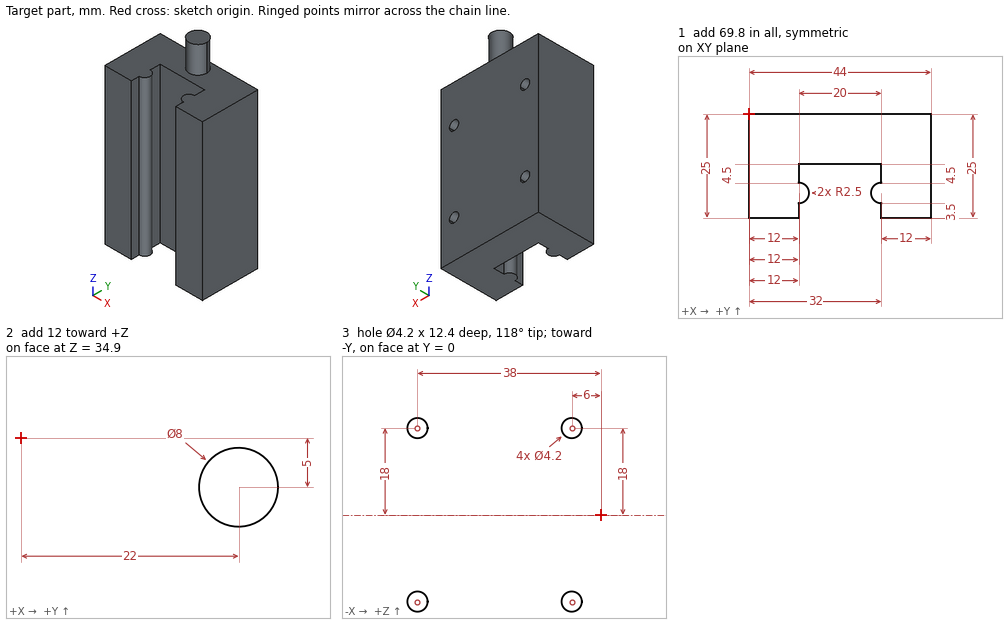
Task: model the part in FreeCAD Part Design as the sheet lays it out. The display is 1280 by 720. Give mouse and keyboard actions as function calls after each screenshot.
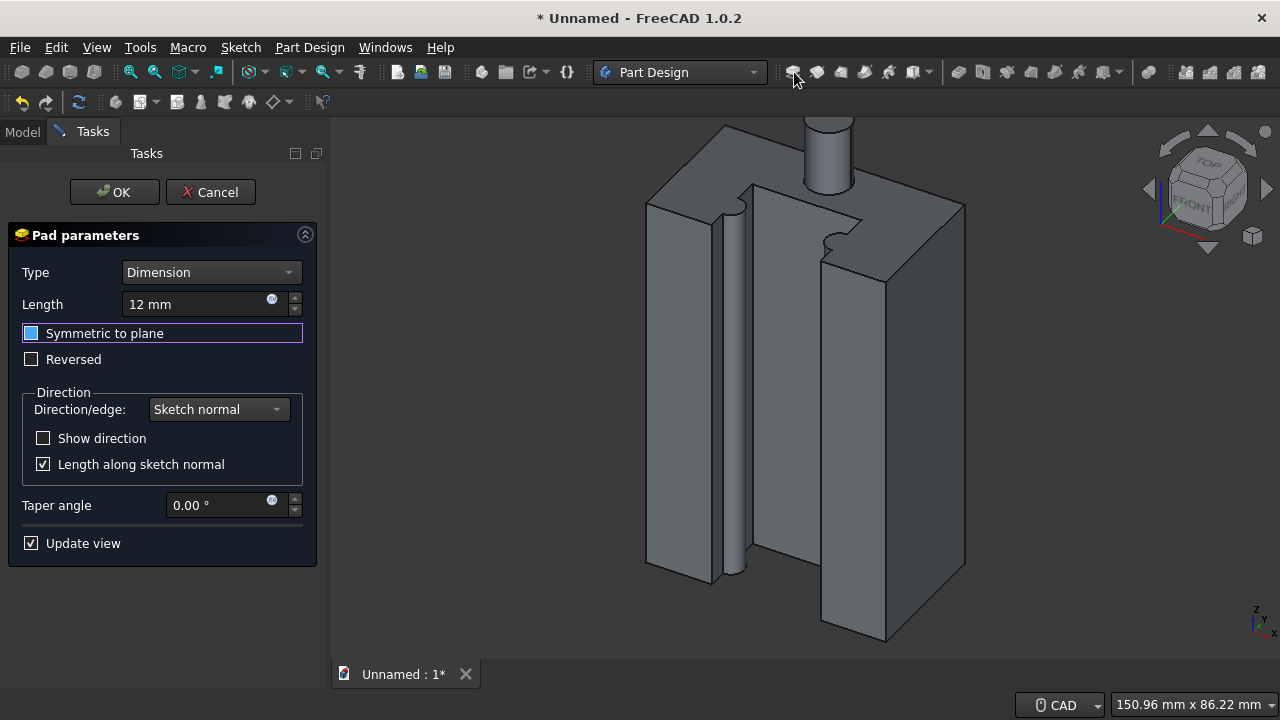
click(115, 192)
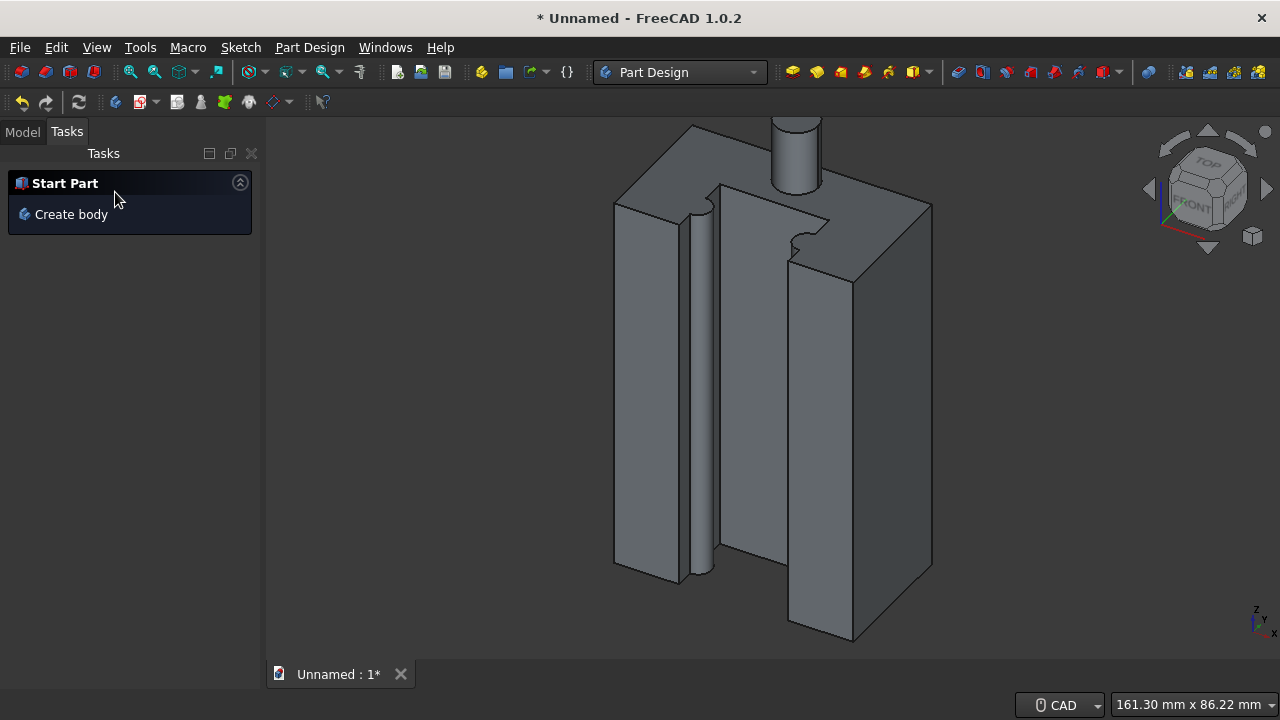
click(132, 72)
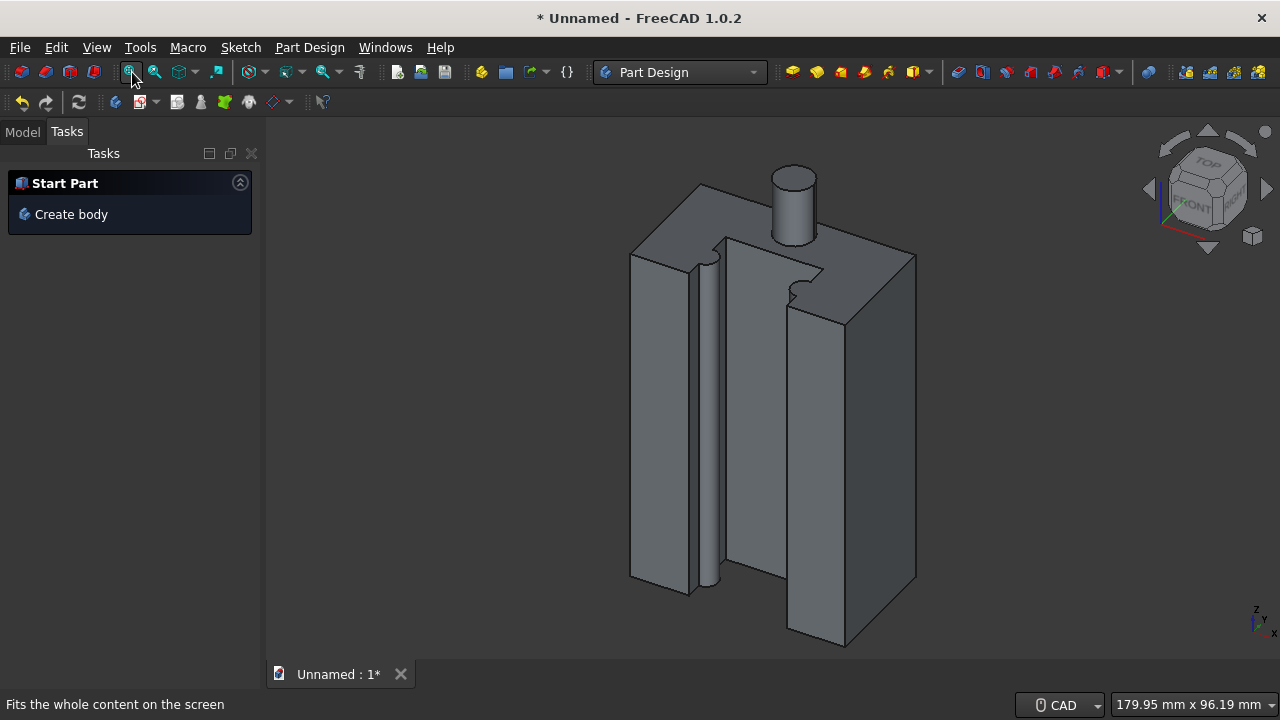
key(4)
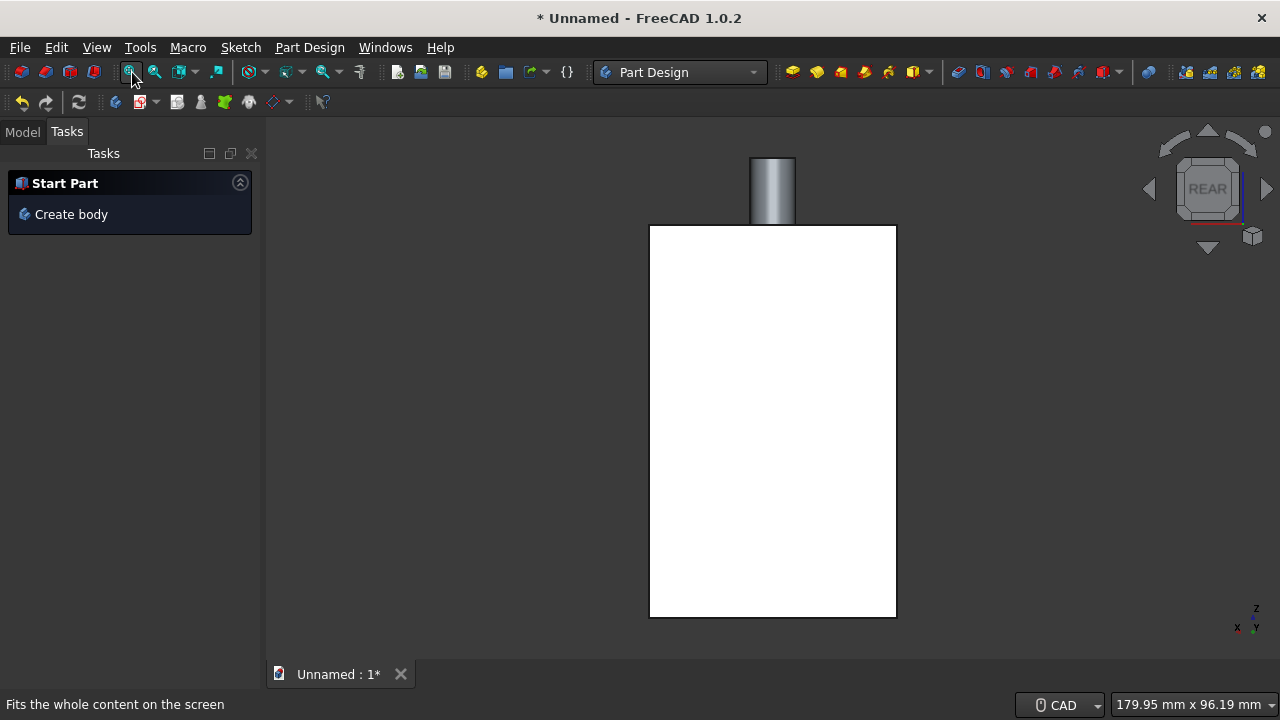
click(773, 365)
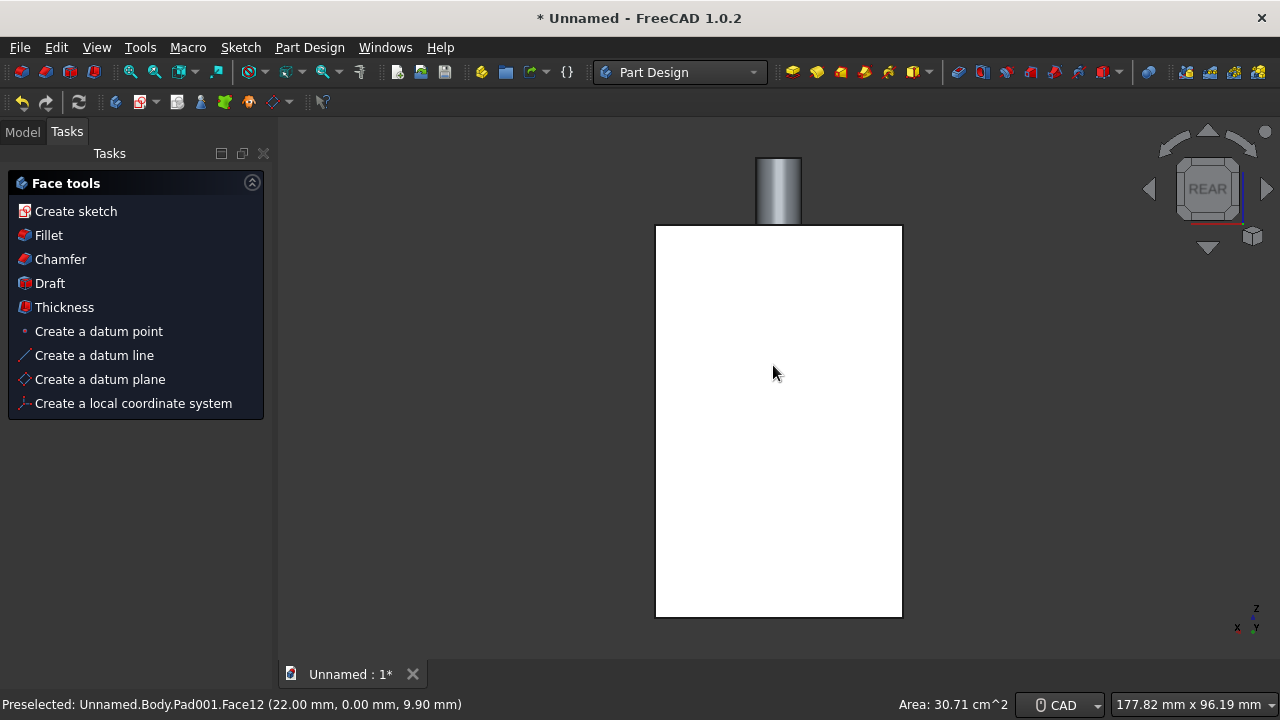
click(140, 102)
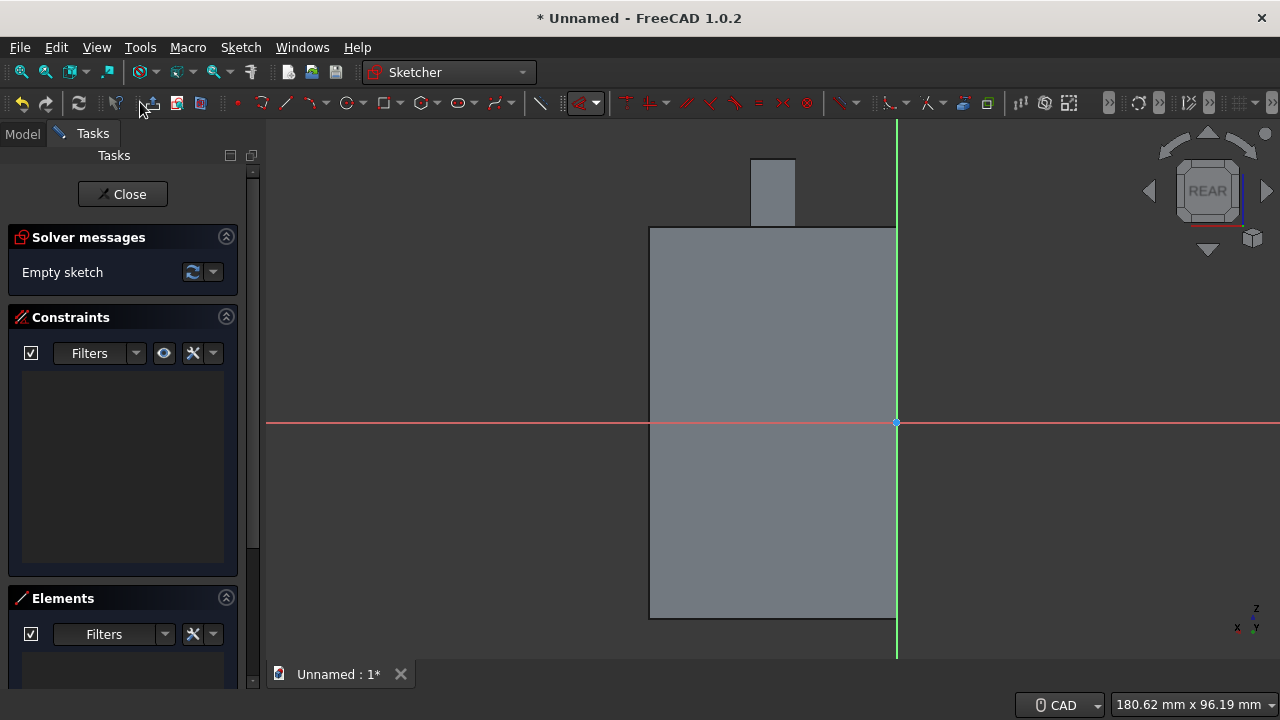
scroll(945, 491, up, 2)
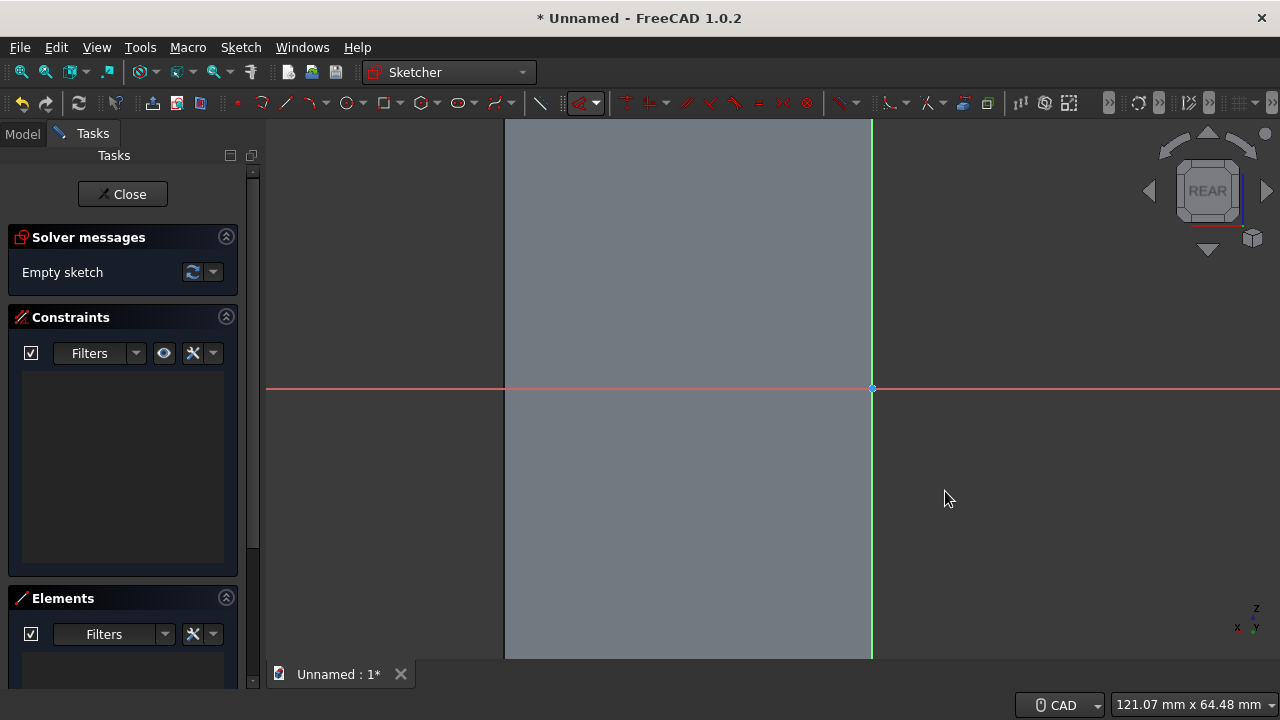
click(348, 104)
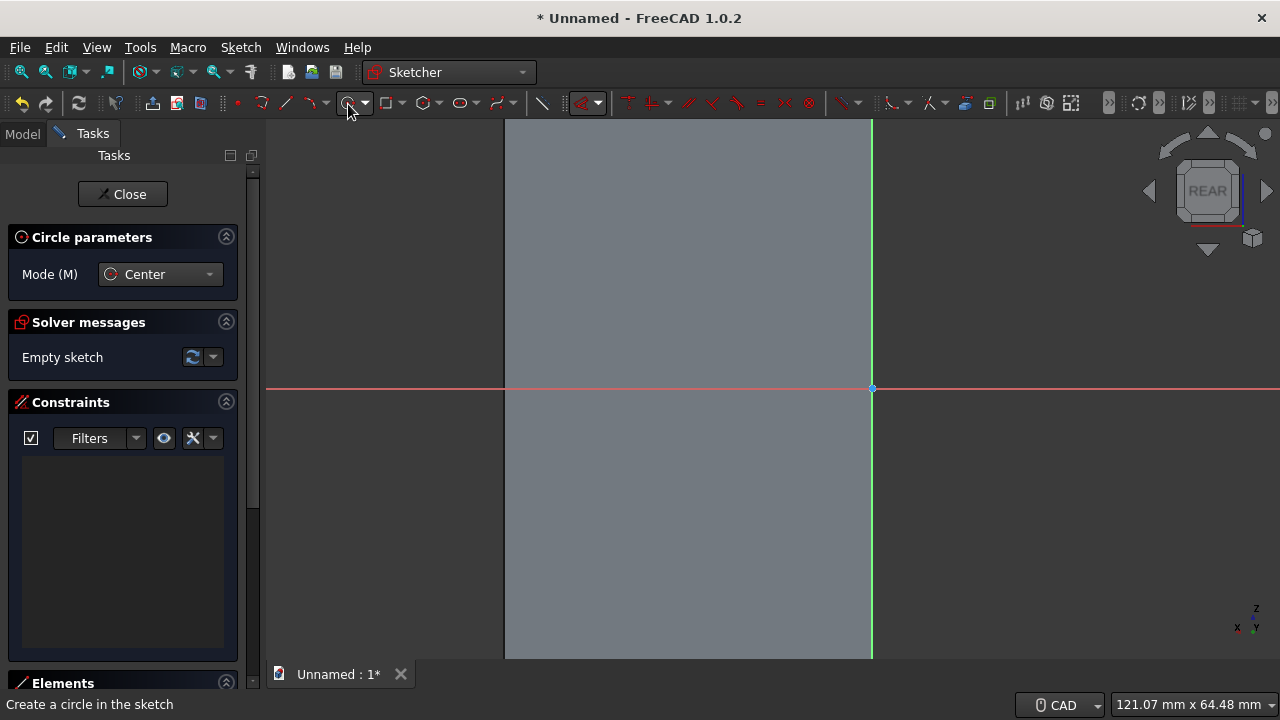
scroll(822, 238, up, 2)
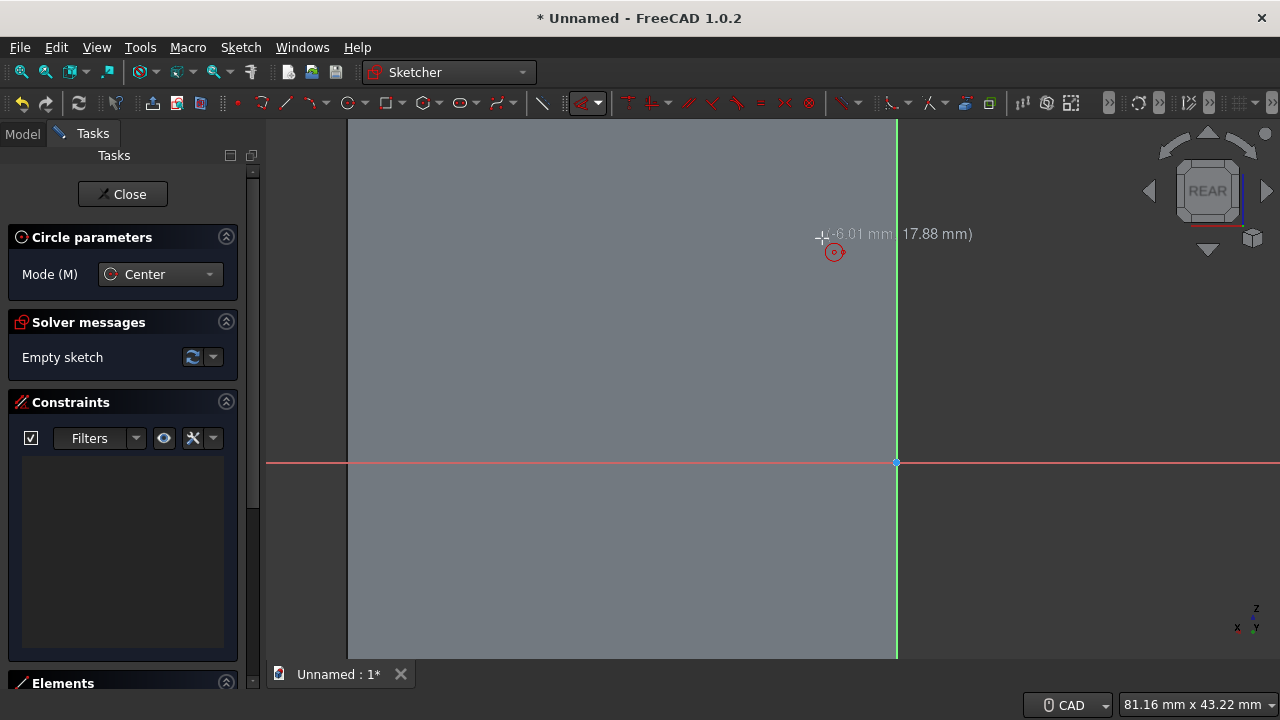
click(822, 238)
click(840, 219)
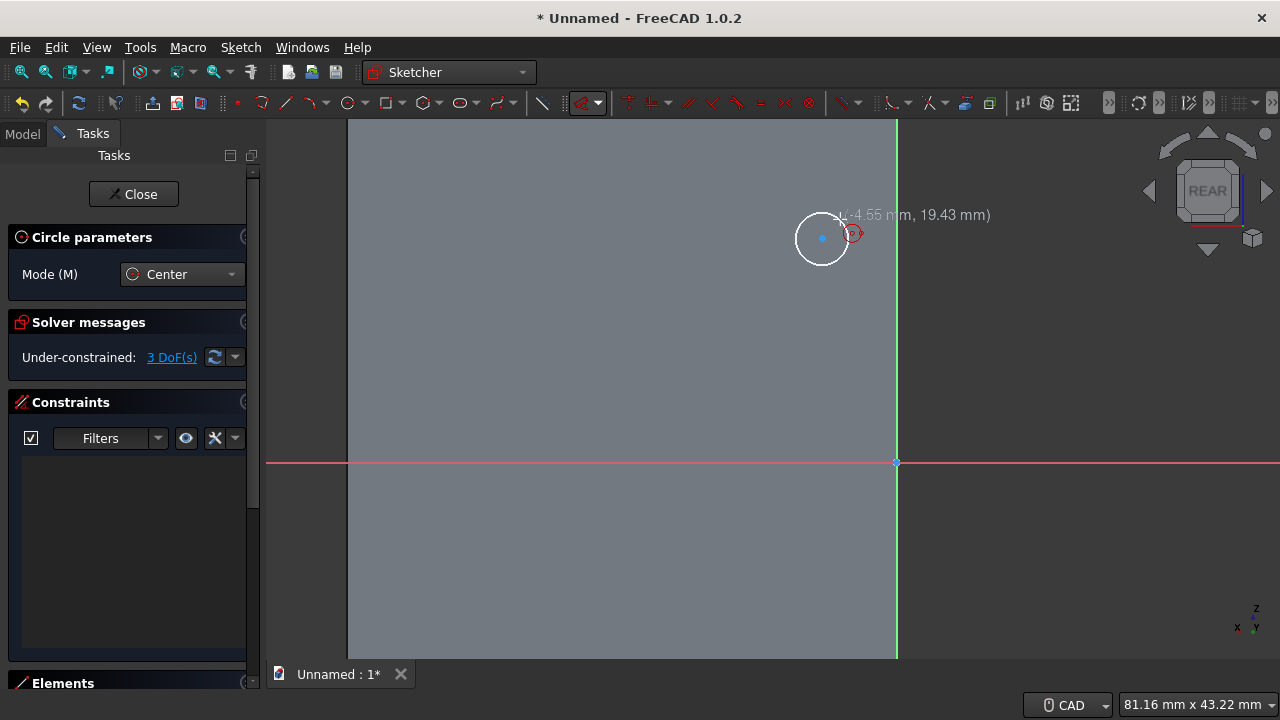
click(422, 238)
click(441, 219)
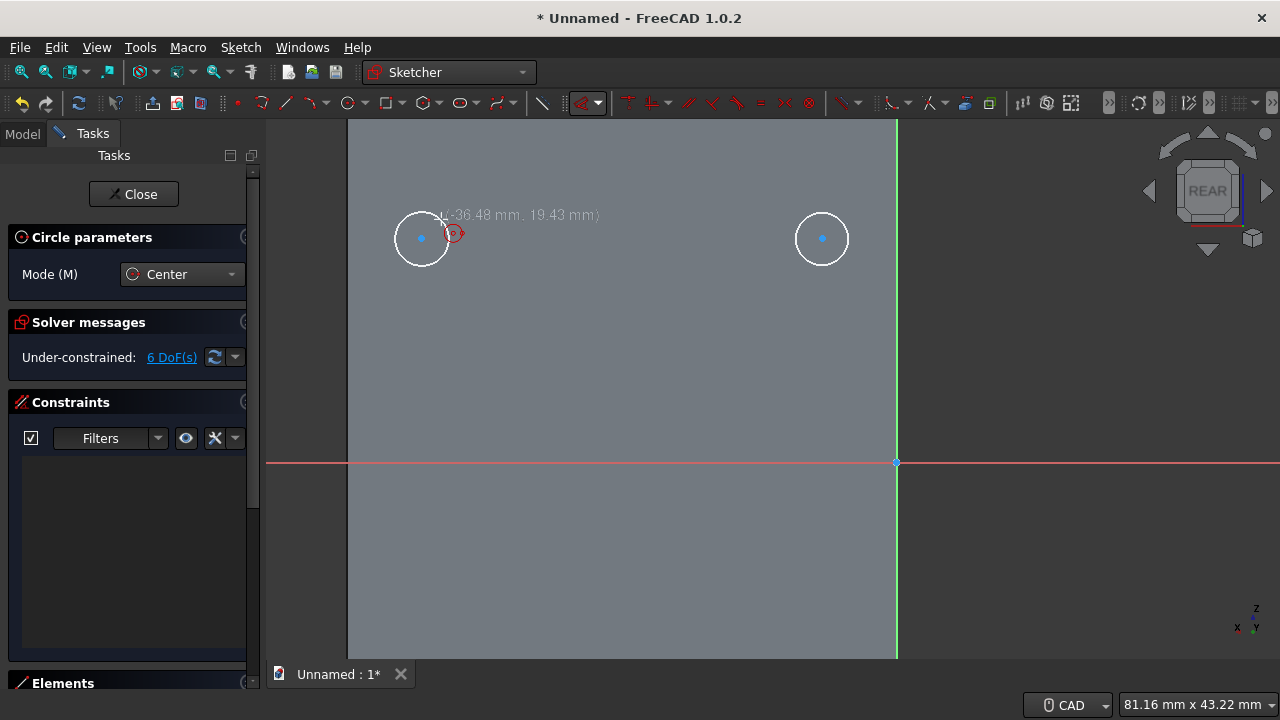
scroll(823, 239, down, 2)